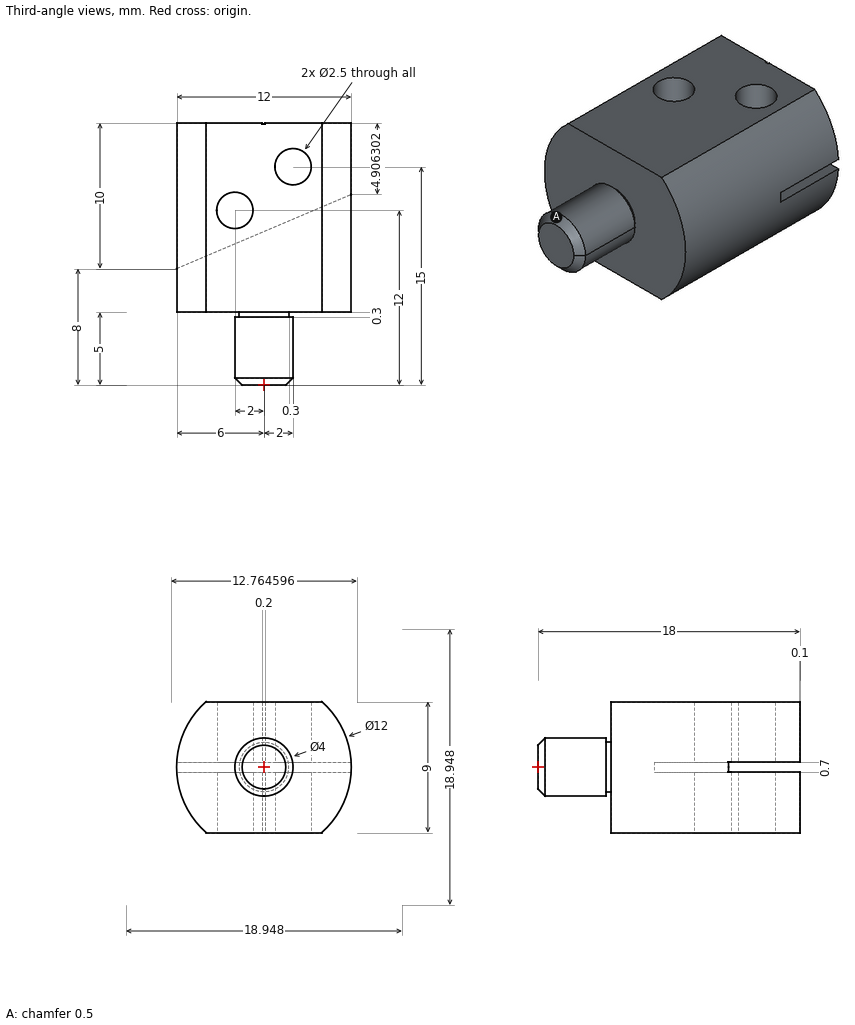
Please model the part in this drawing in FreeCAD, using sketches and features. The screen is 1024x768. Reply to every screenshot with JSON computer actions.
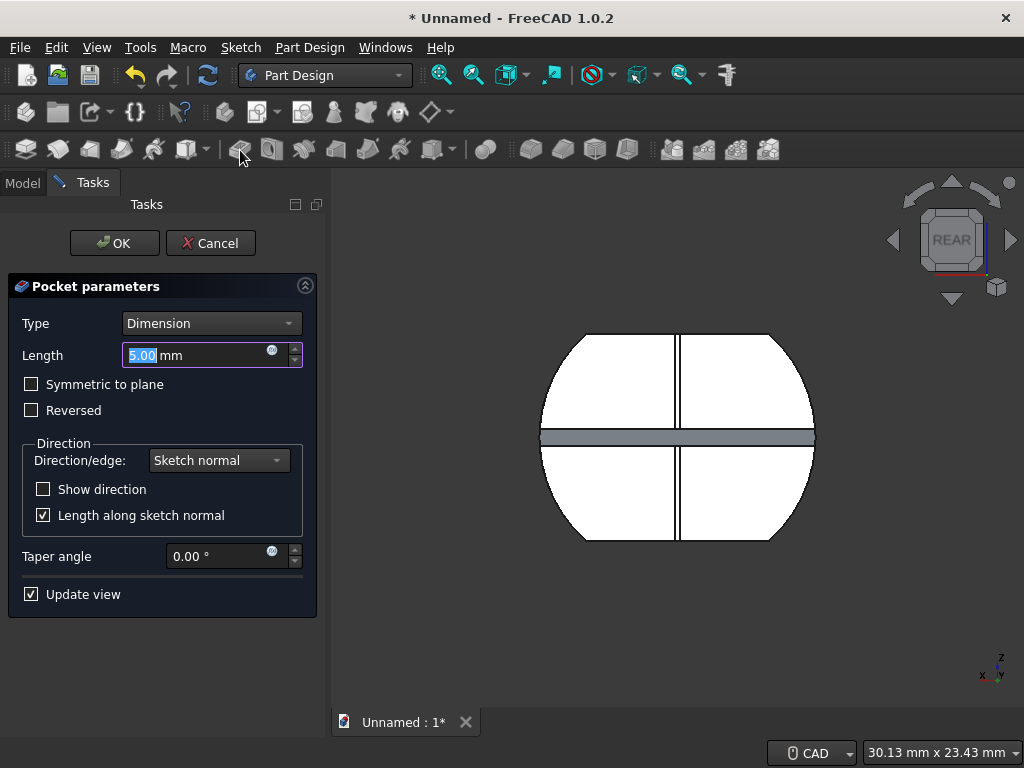
{"action": "type", "text": "0.1"}
{"action": "key", "text": "Tab"}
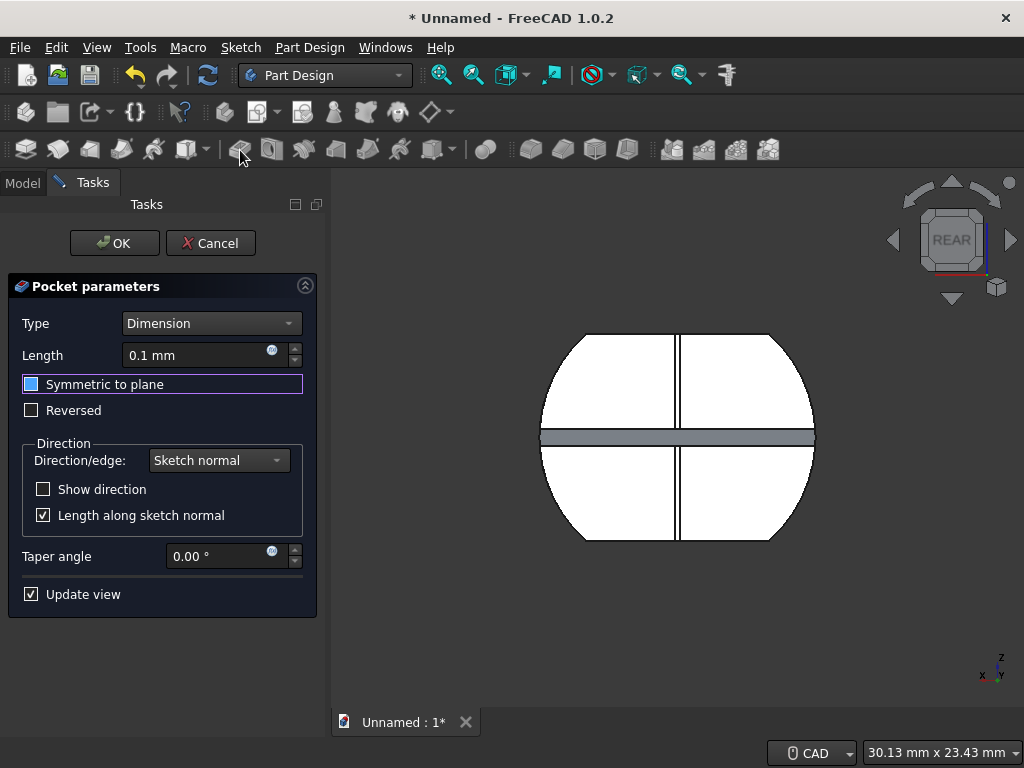
{"action": "left_click", "coordinate": [115, 243]}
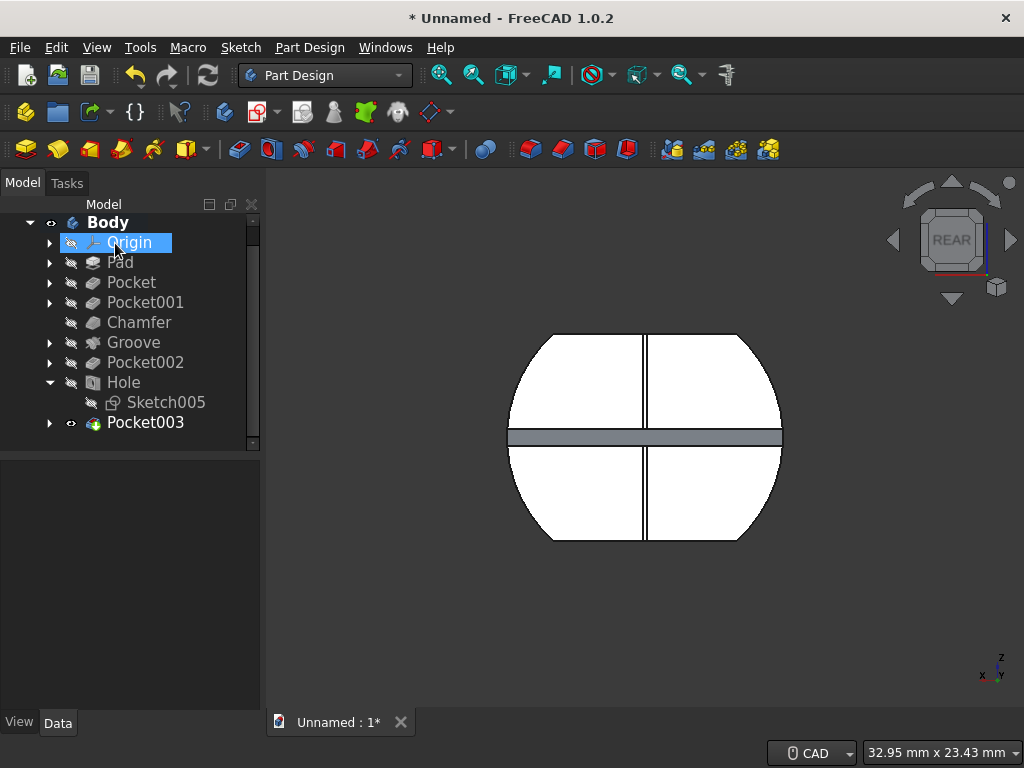
{"action": "key", "text": "0"}